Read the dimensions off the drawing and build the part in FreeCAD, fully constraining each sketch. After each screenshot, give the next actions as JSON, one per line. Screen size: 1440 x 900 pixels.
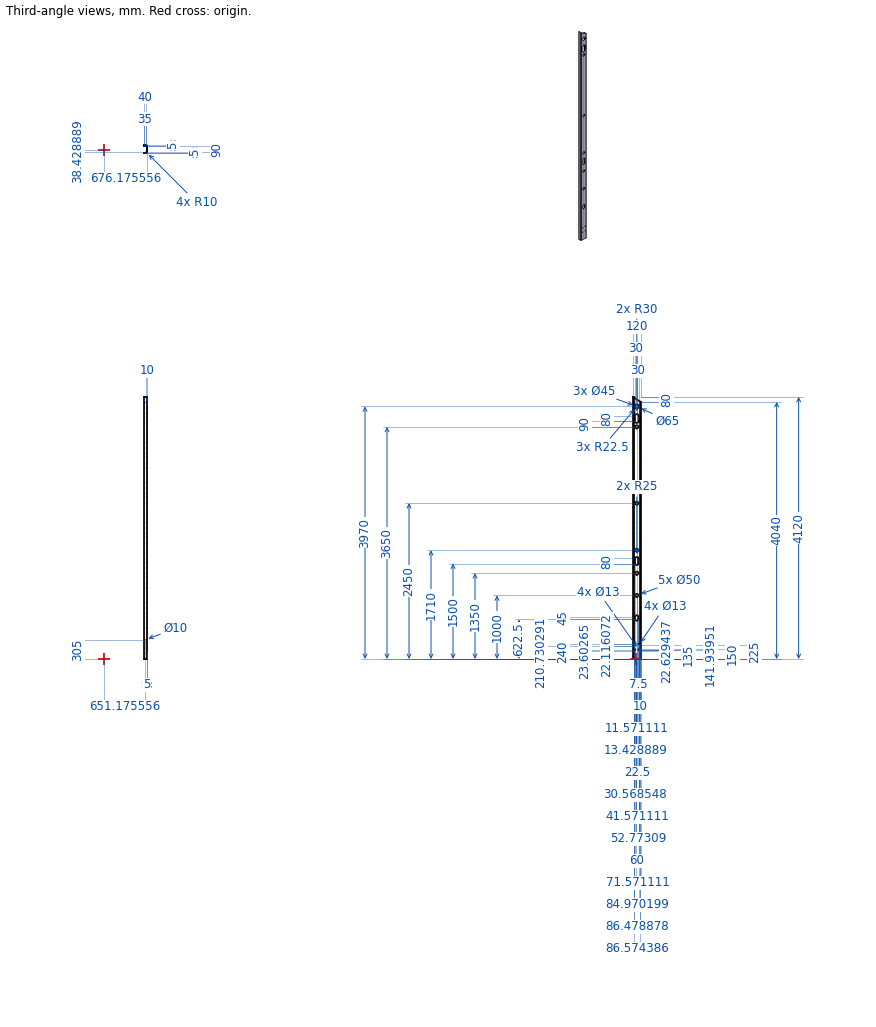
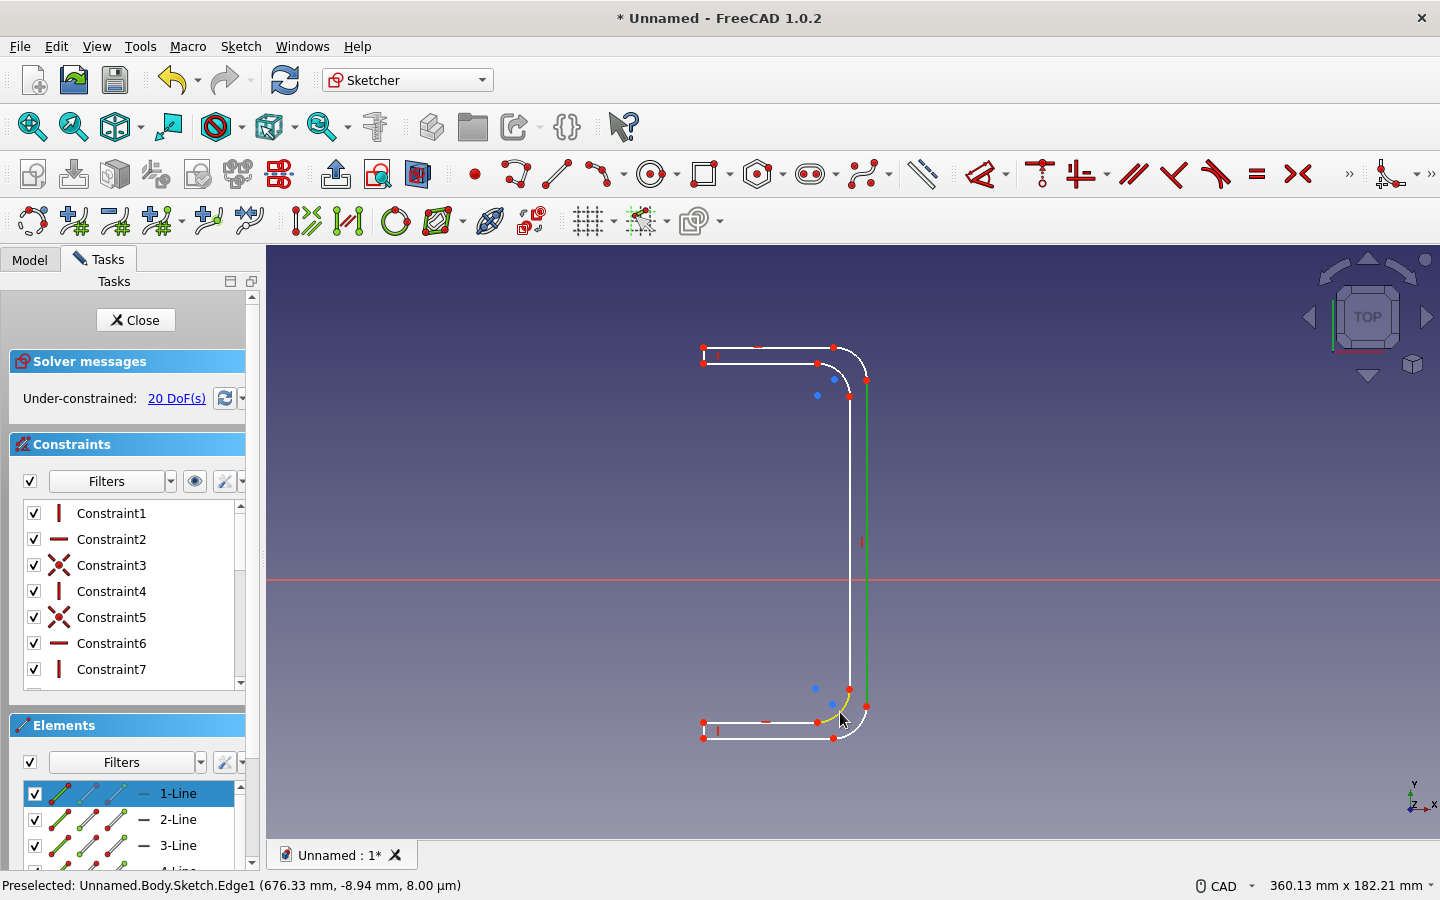
{"action": "left_click", "coordinate": [863, 366]}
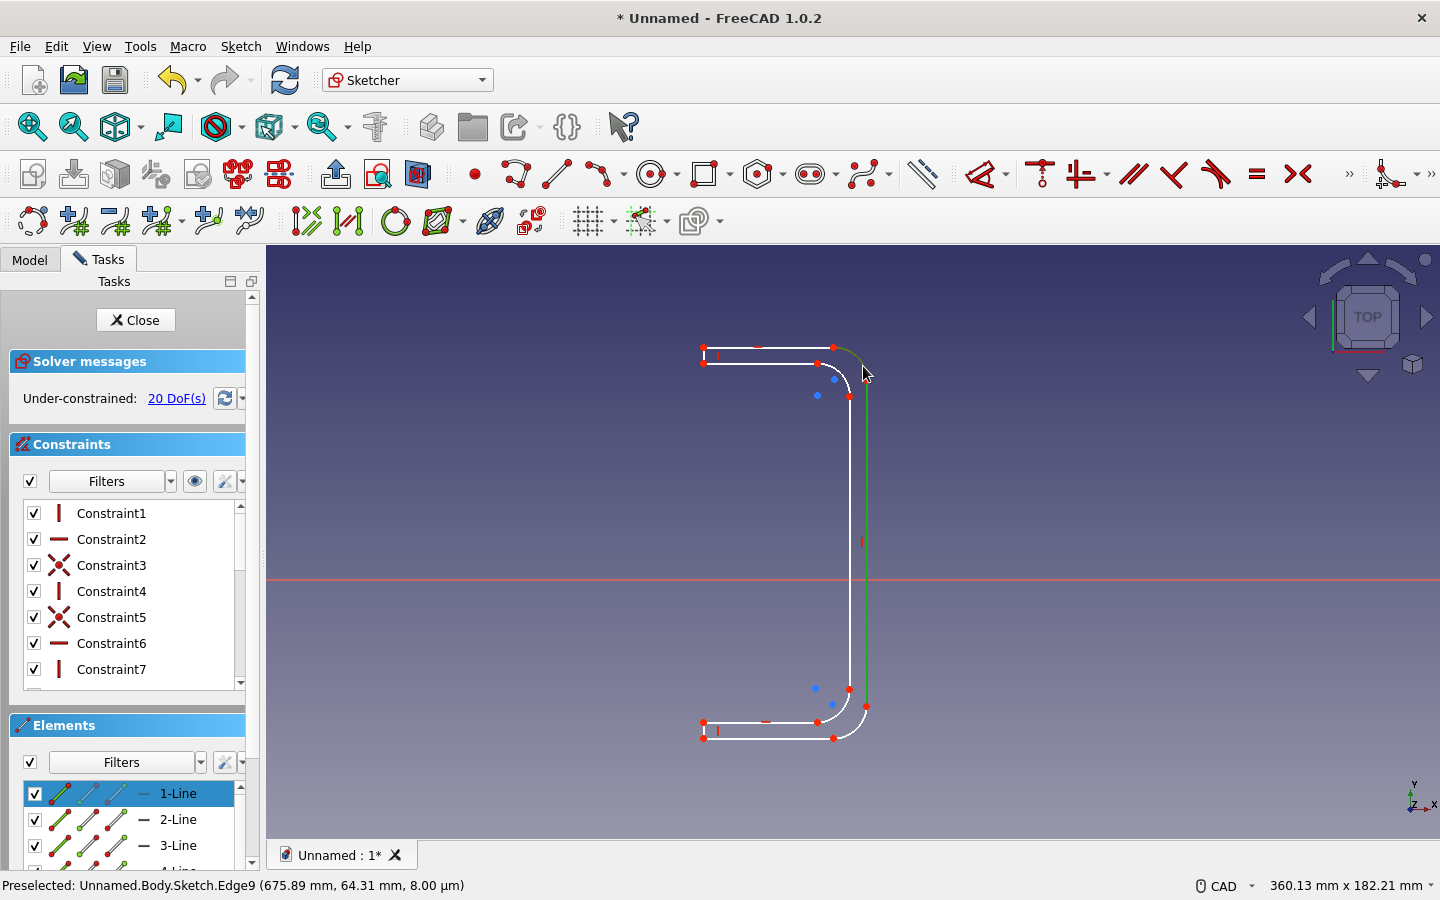
{"action": "key", "text": "t"}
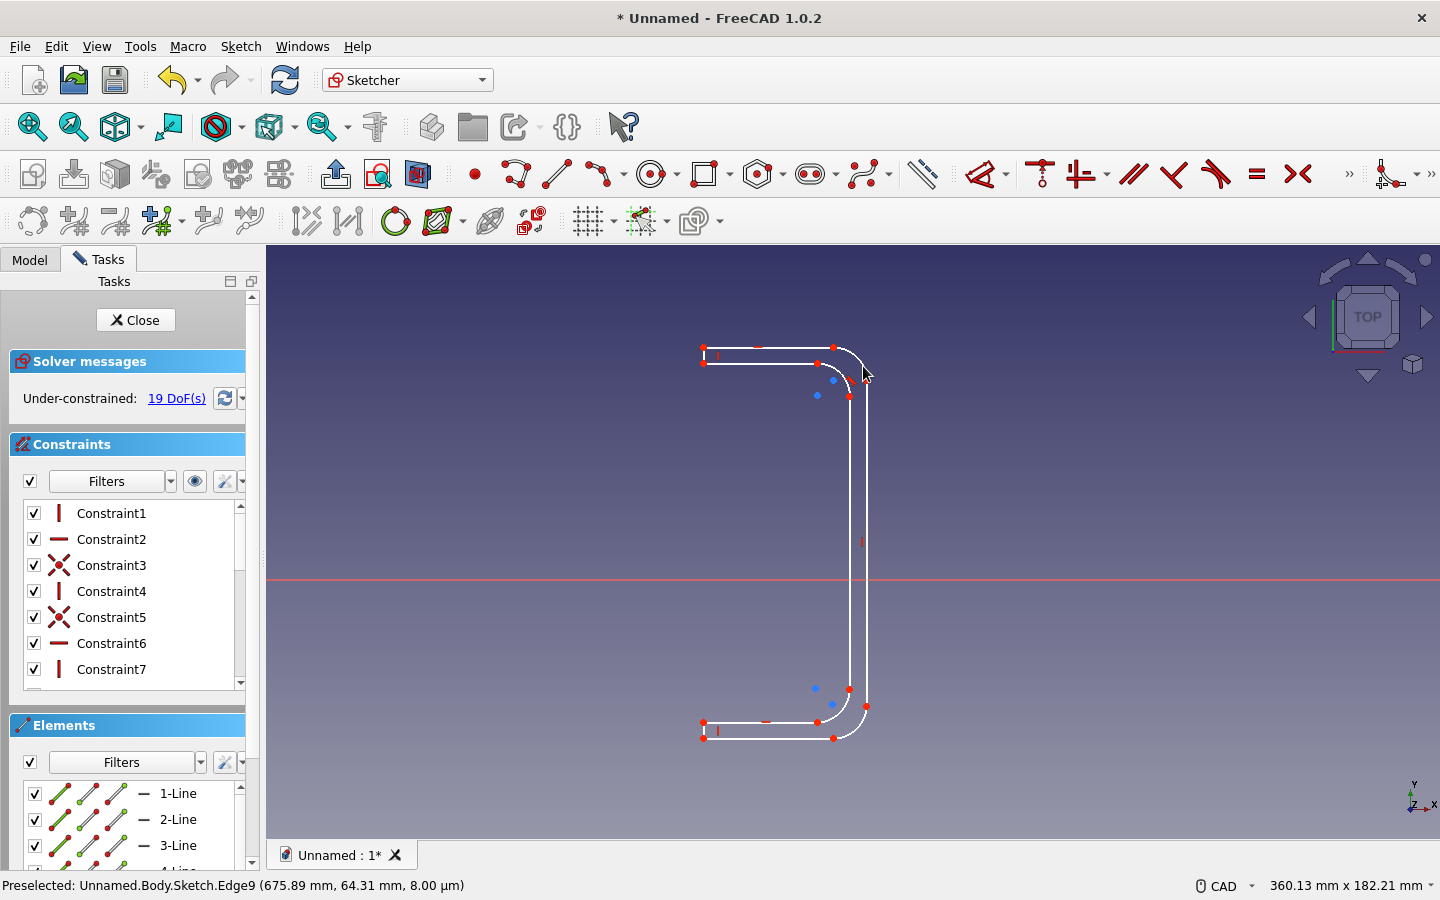
{"action": "left_click", "coordinate": [867, 609]}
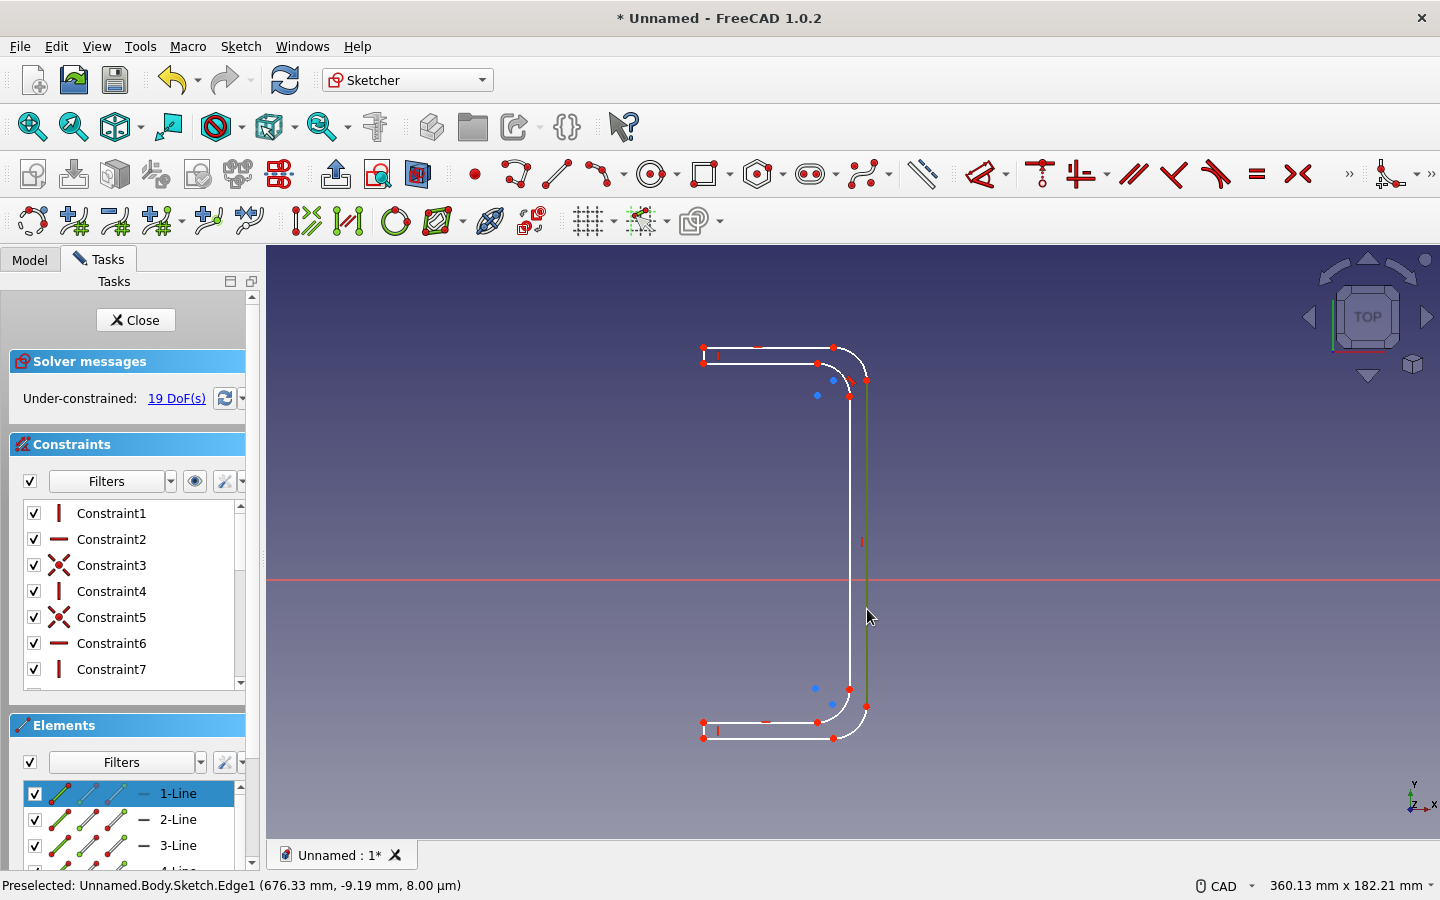
{"action": "left_click", "coordinate": [848, 735]}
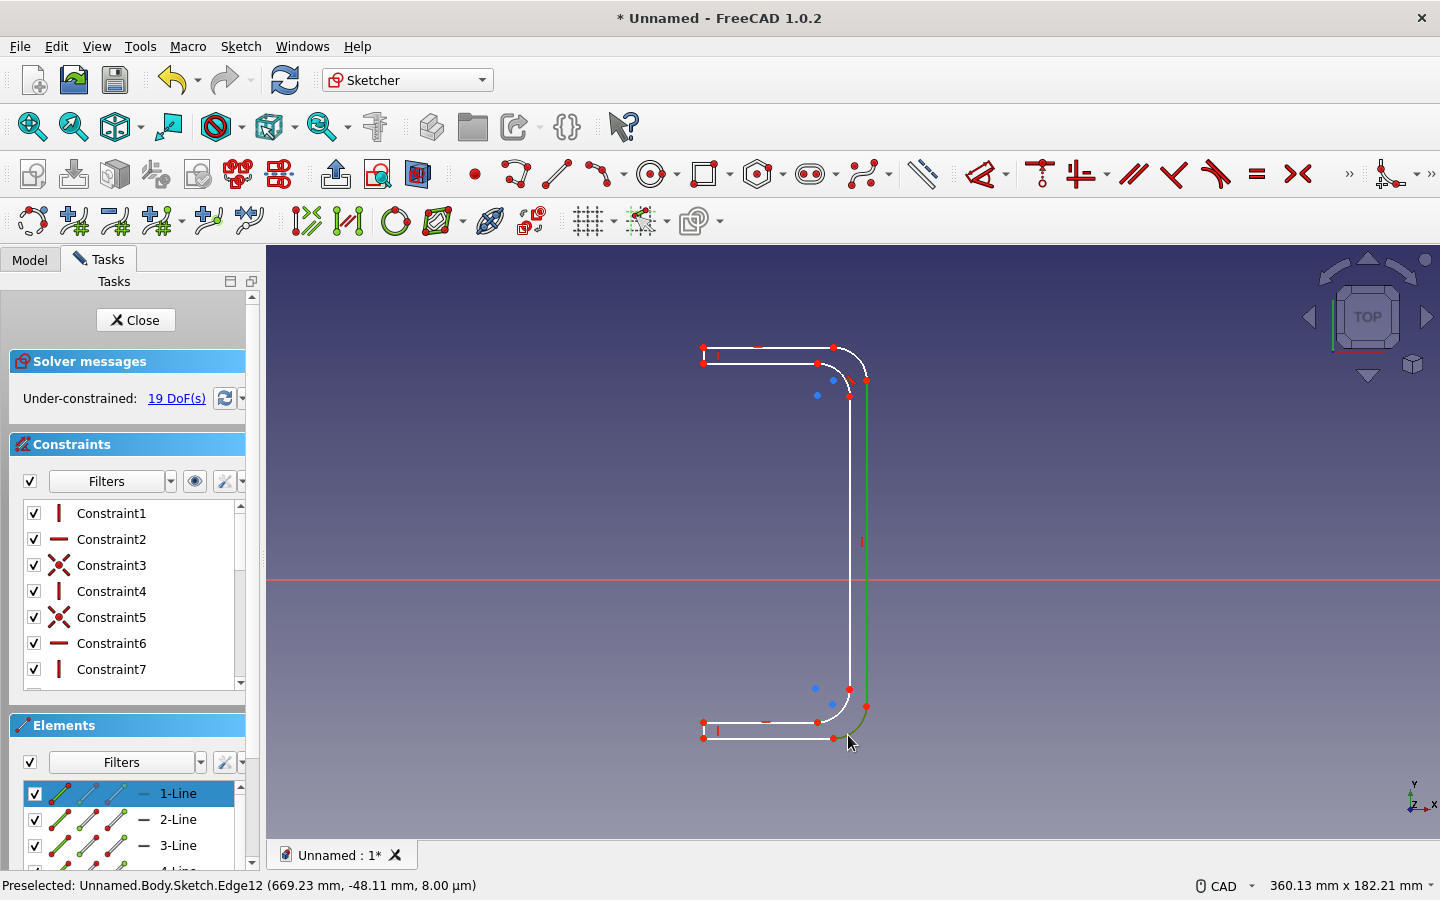
{"action": "key", "text": "t"}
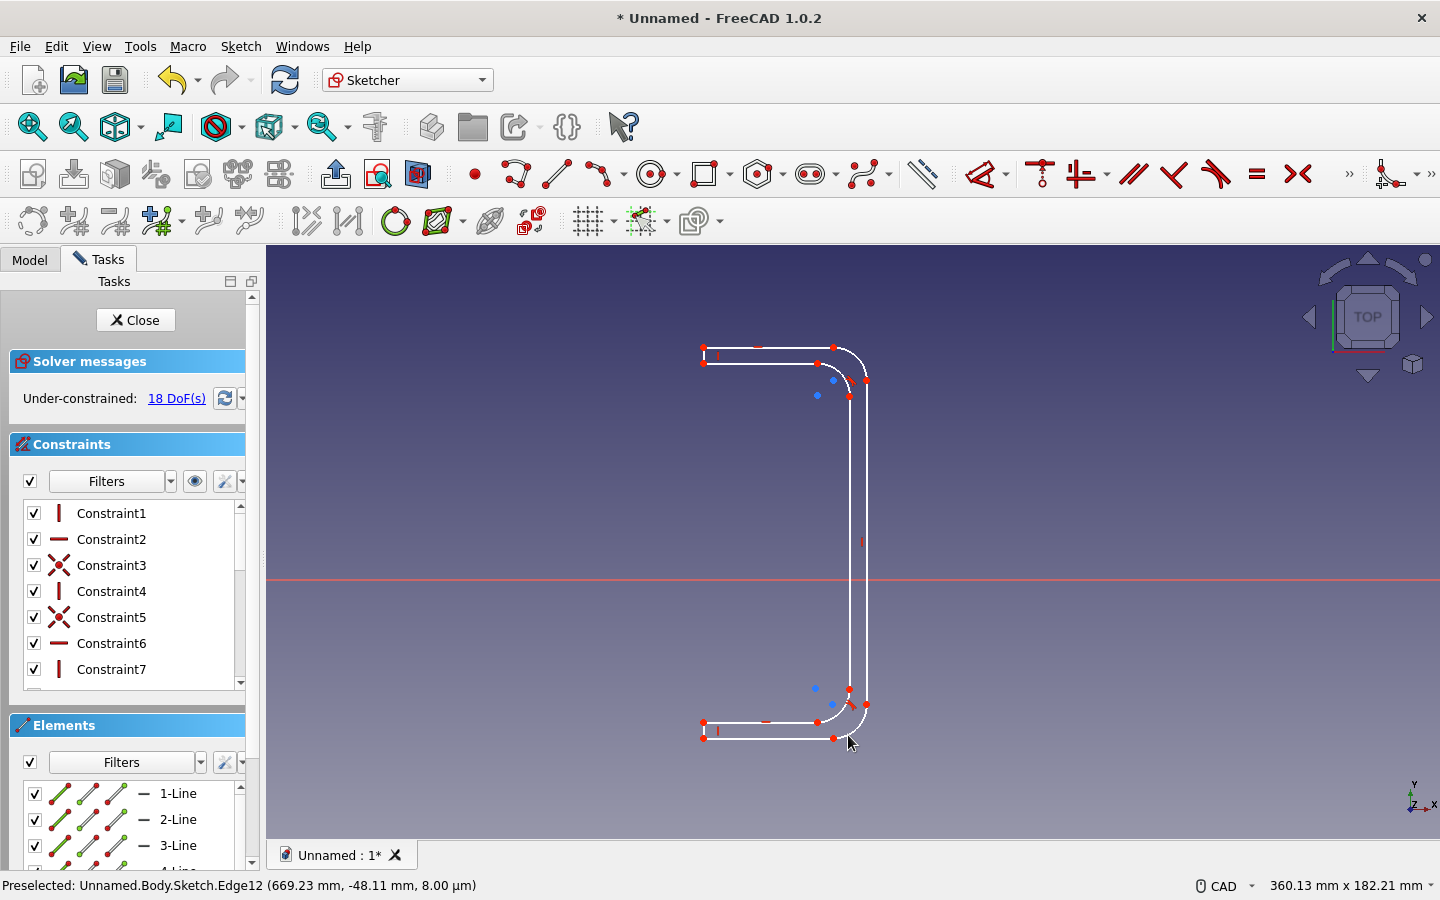
{"action": "left_click", "coordinate": [795, 348]}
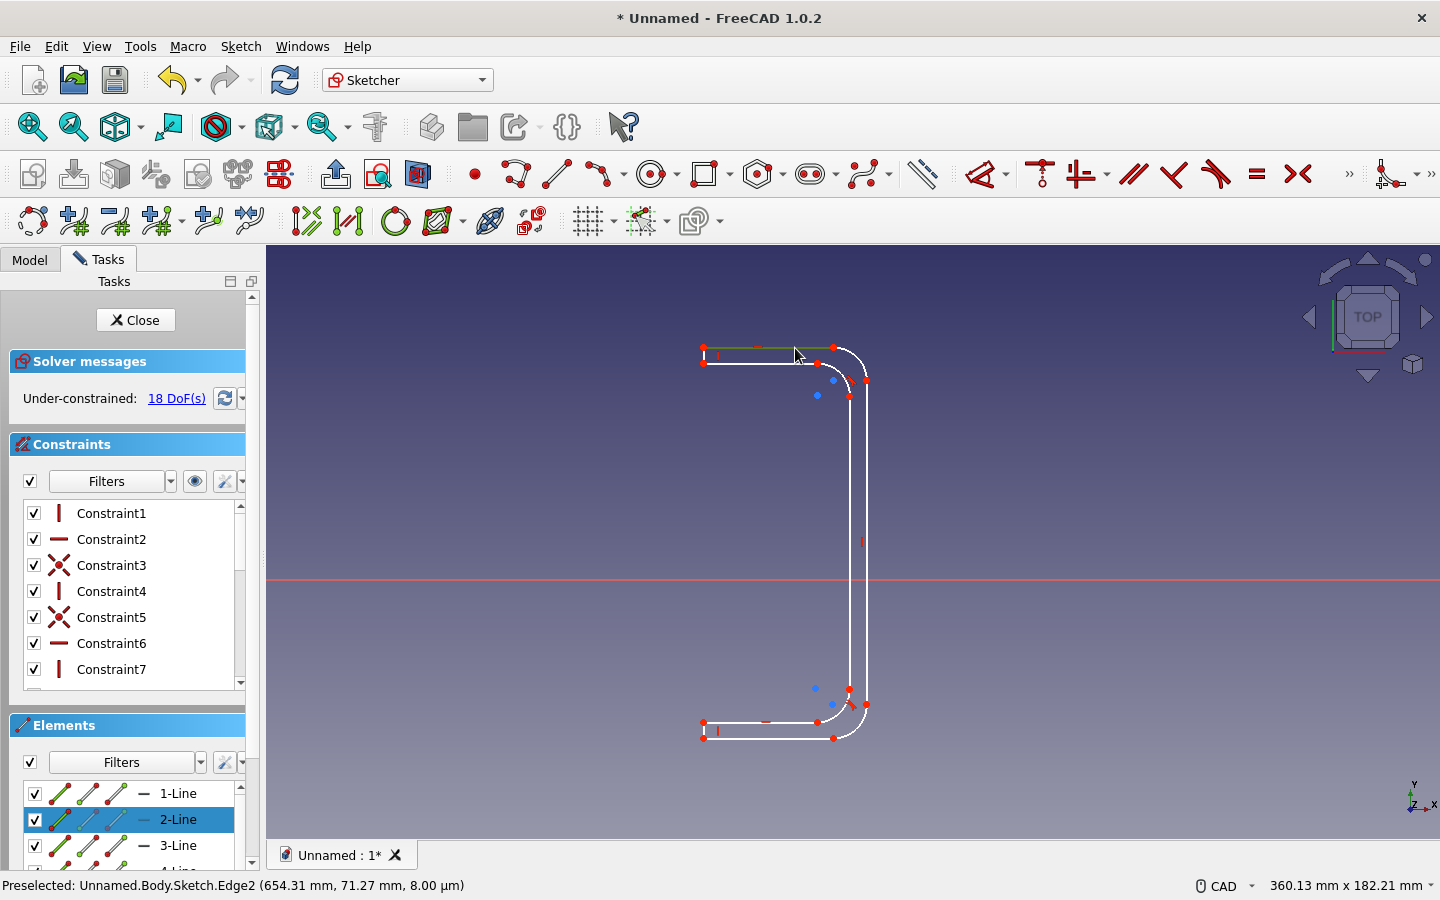
{"action": "left_click", "coordinate": [863, 366]}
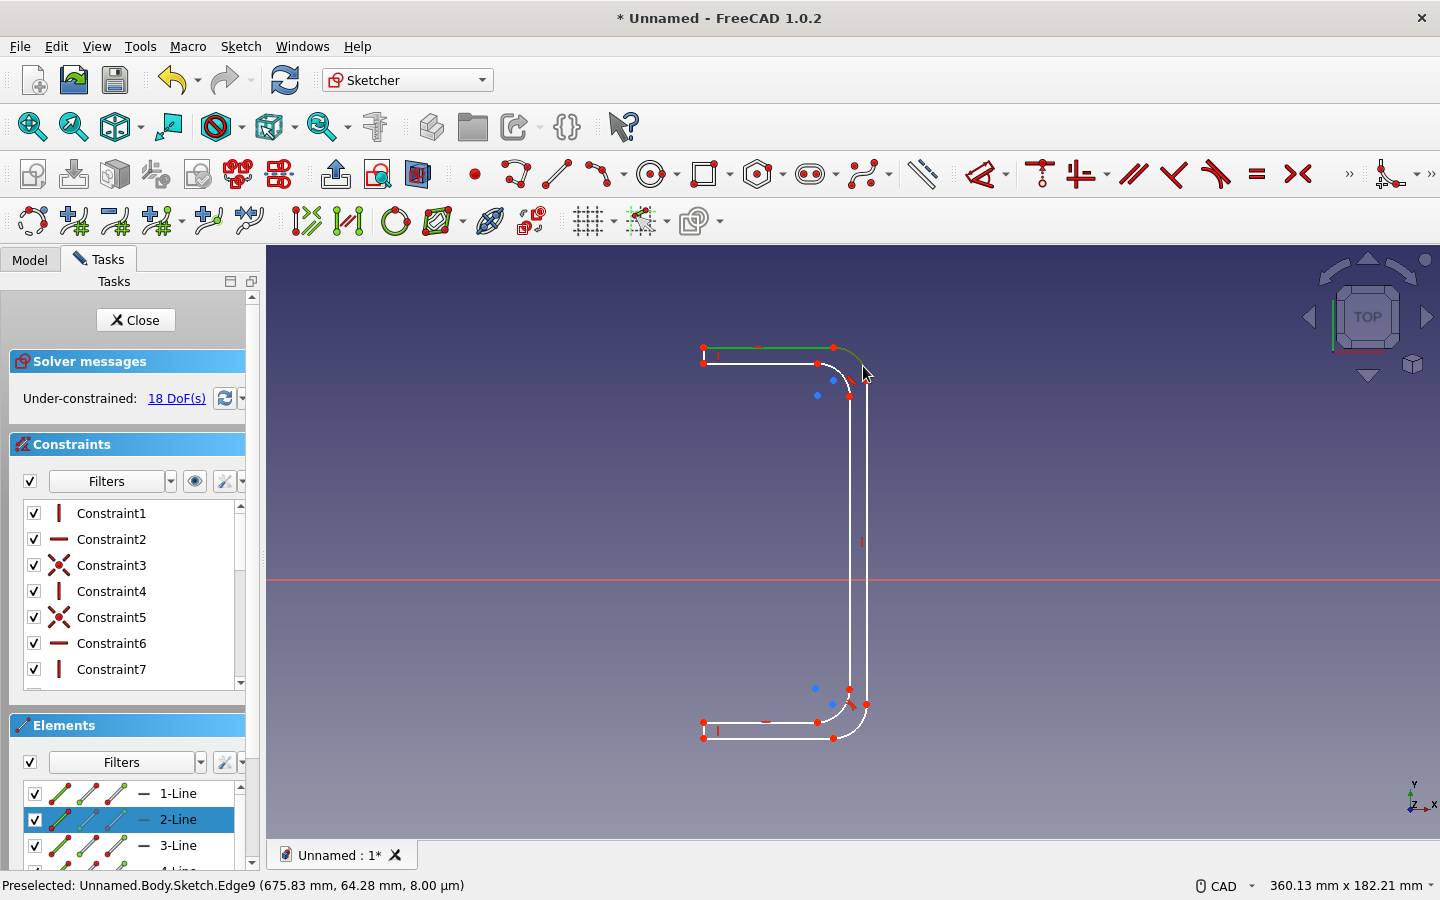
{"action": "key", "text": "t"}